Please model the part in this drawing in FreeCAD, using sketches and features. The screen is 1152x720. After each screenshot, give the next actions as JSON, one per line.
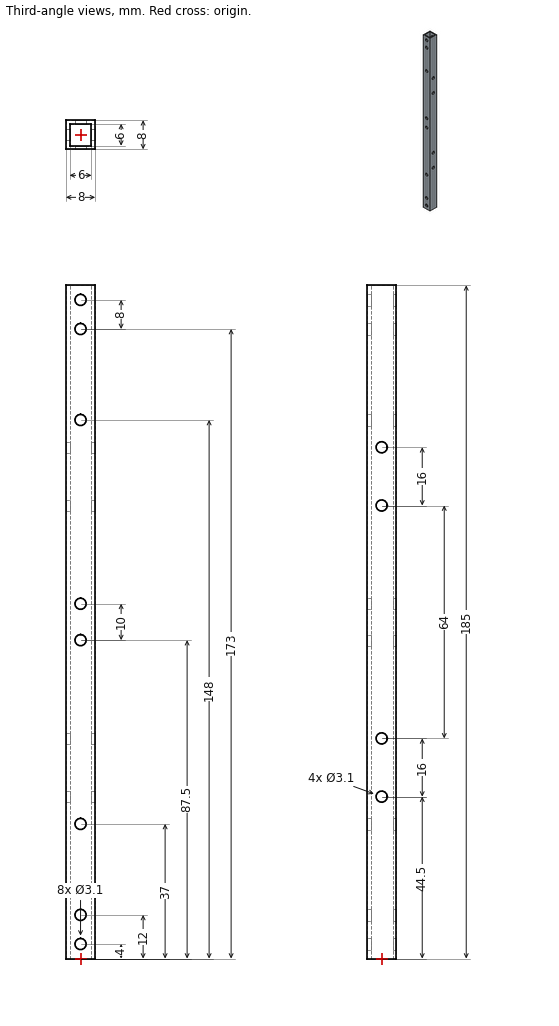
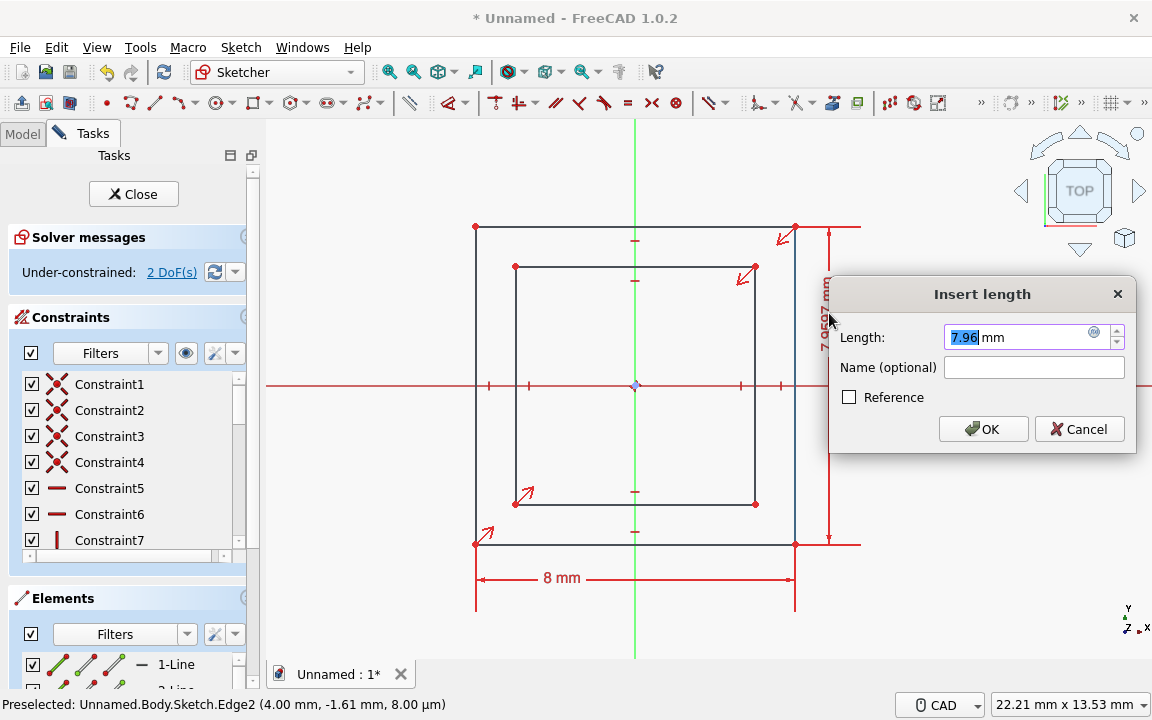
{"action": "type", "text": "8"}
{"action": "key", "text": "Return"}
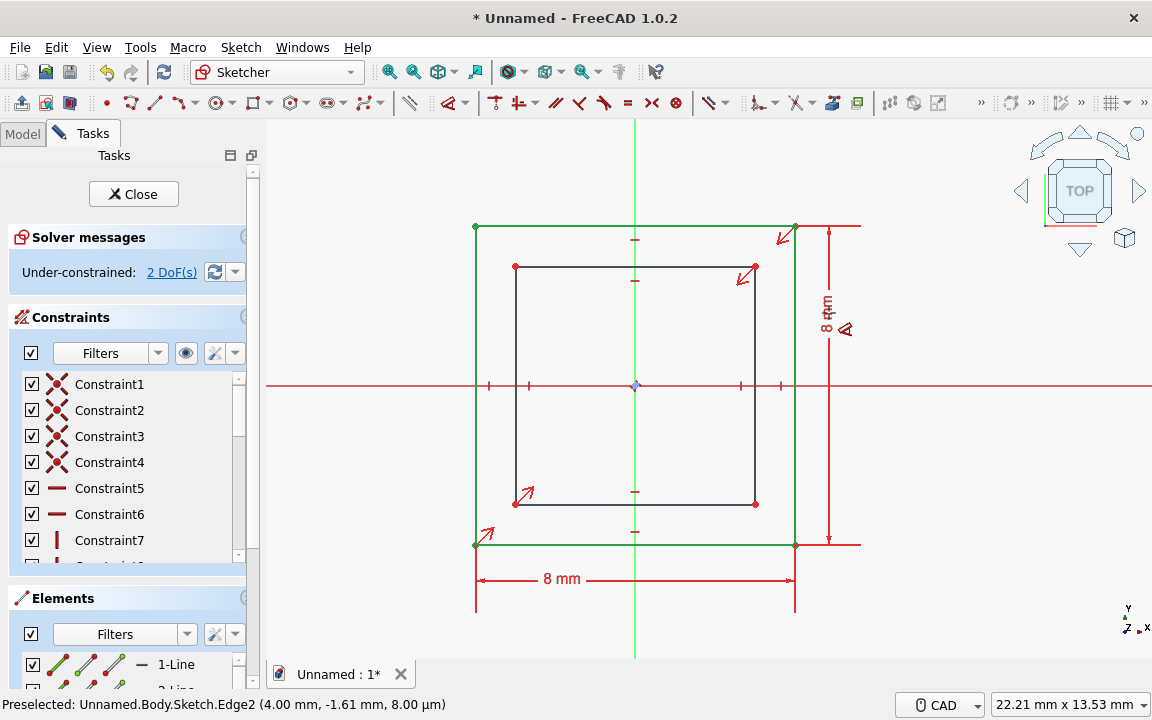
{"action": "left_click", "coordinate": [588, 505]}
{"action": "left_click", "coordinate": [580, 471]}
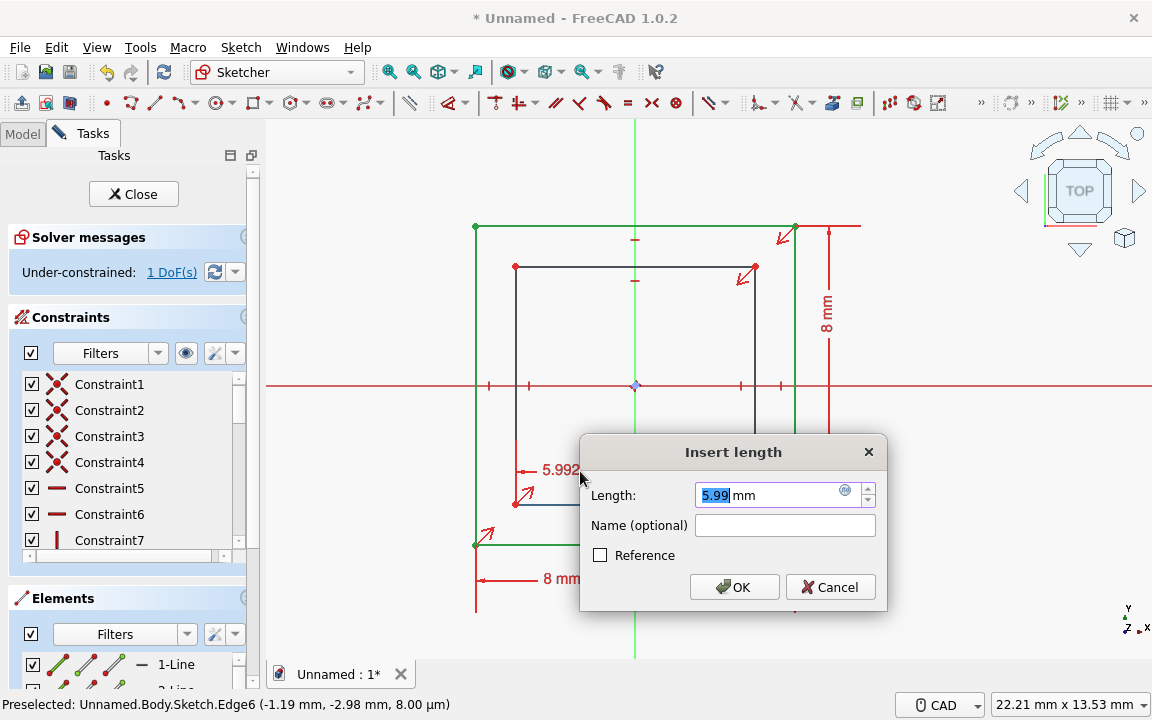
{"action": "type", "text": "6"}
{"action": "key", "text": "Return"}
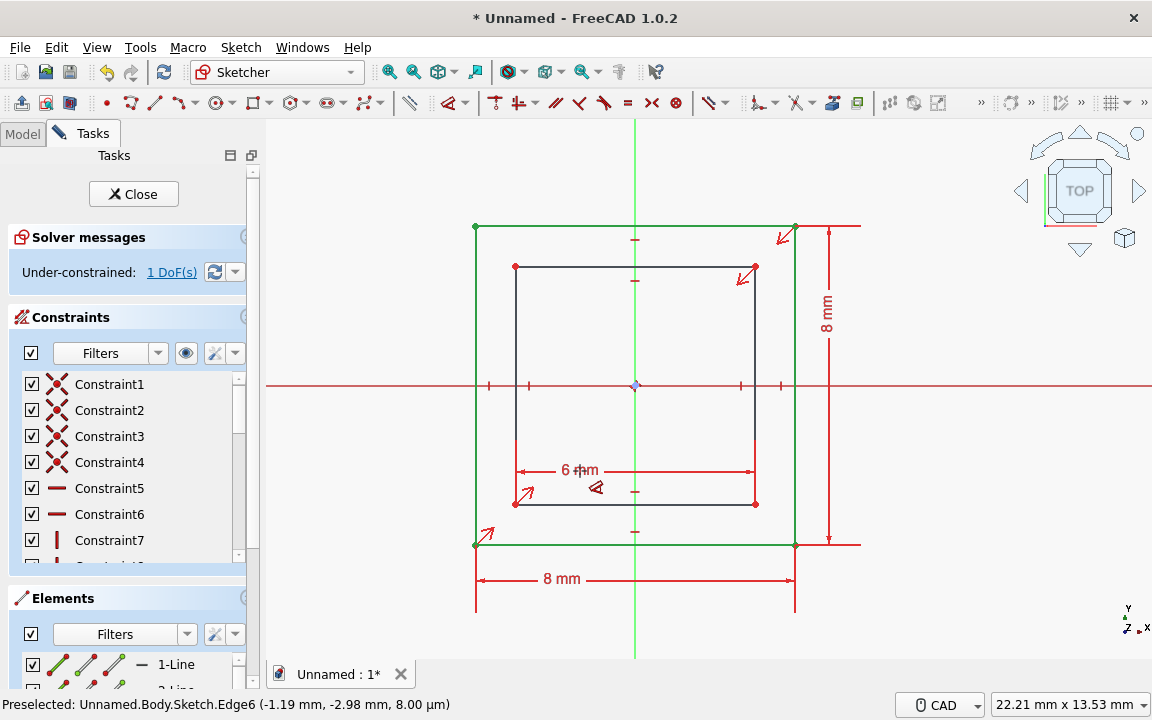
{"action": "left_click", "coordinate": [755, 433]}
{"action": "left_click", "coordinate": [721, 331]}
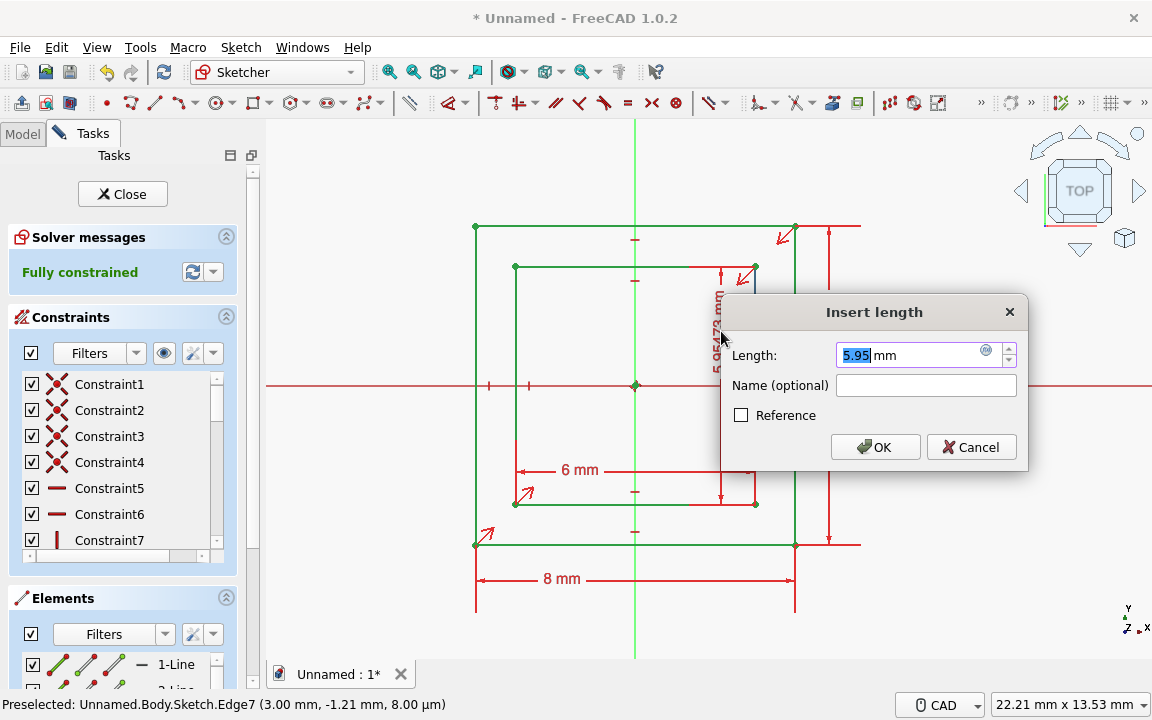
{"action": "type", "text": "6"}
{"action": "key", "text": "Return"}
{"action": "key", "text": "Escape"}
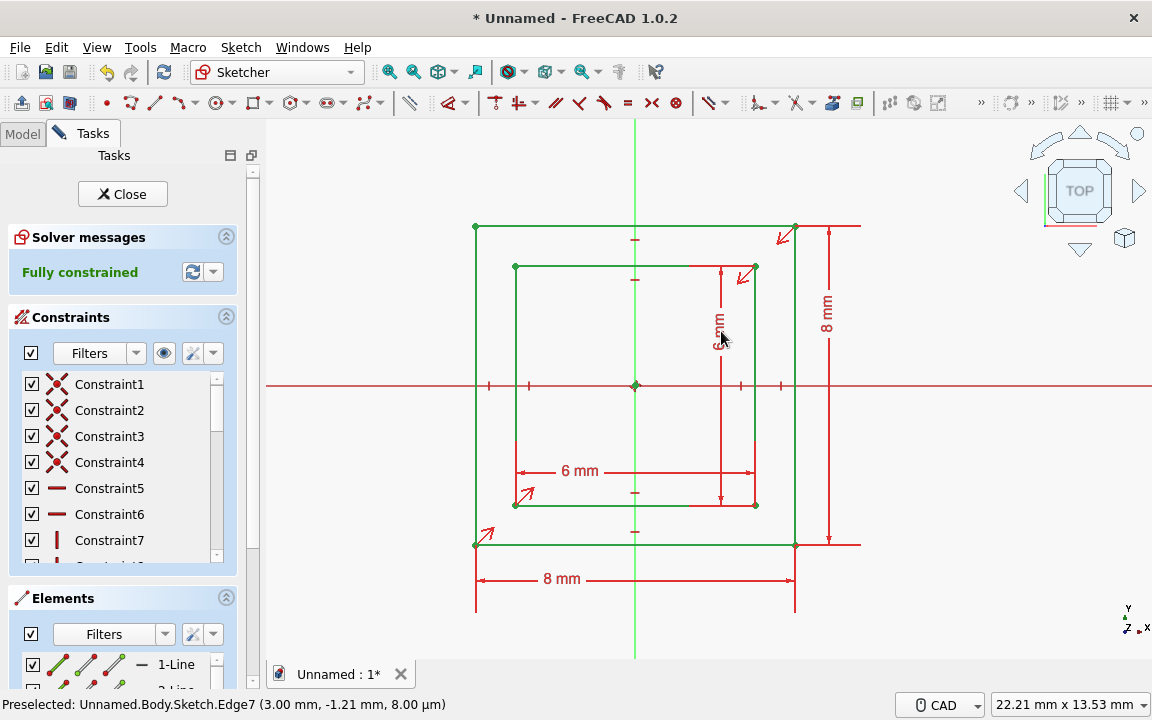
{"action": "left_click", "coordinate": [123, 194]}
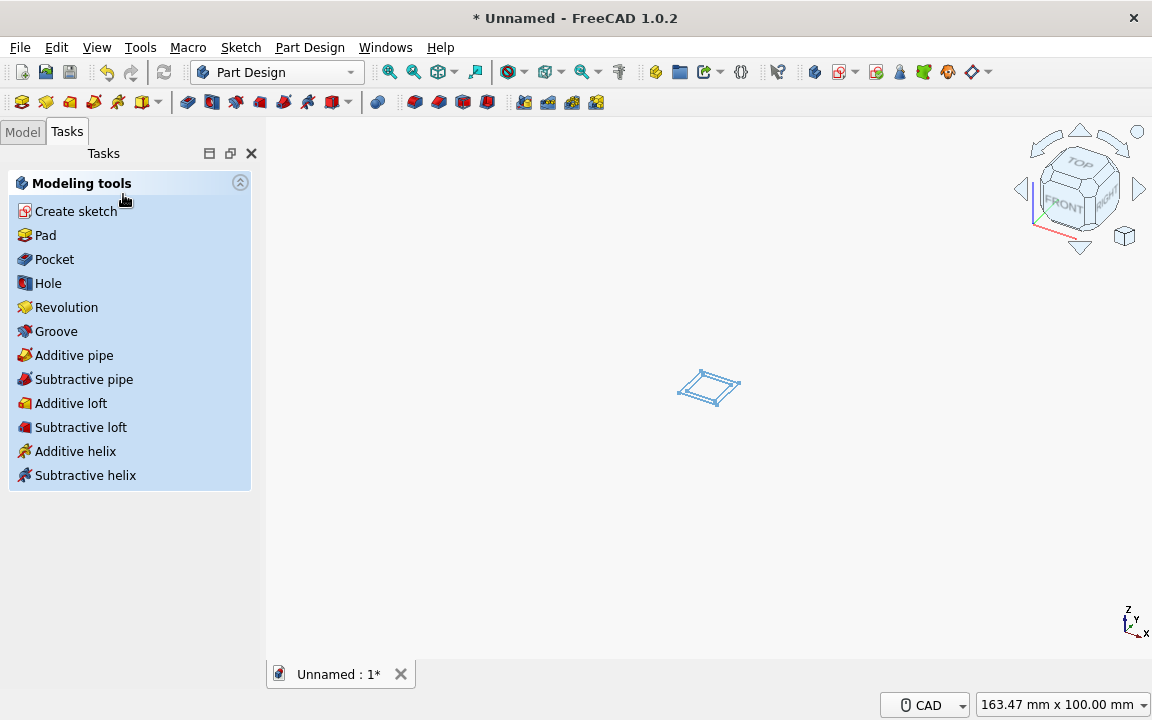
{"action": "left_click", "coordinate": [22, 102]}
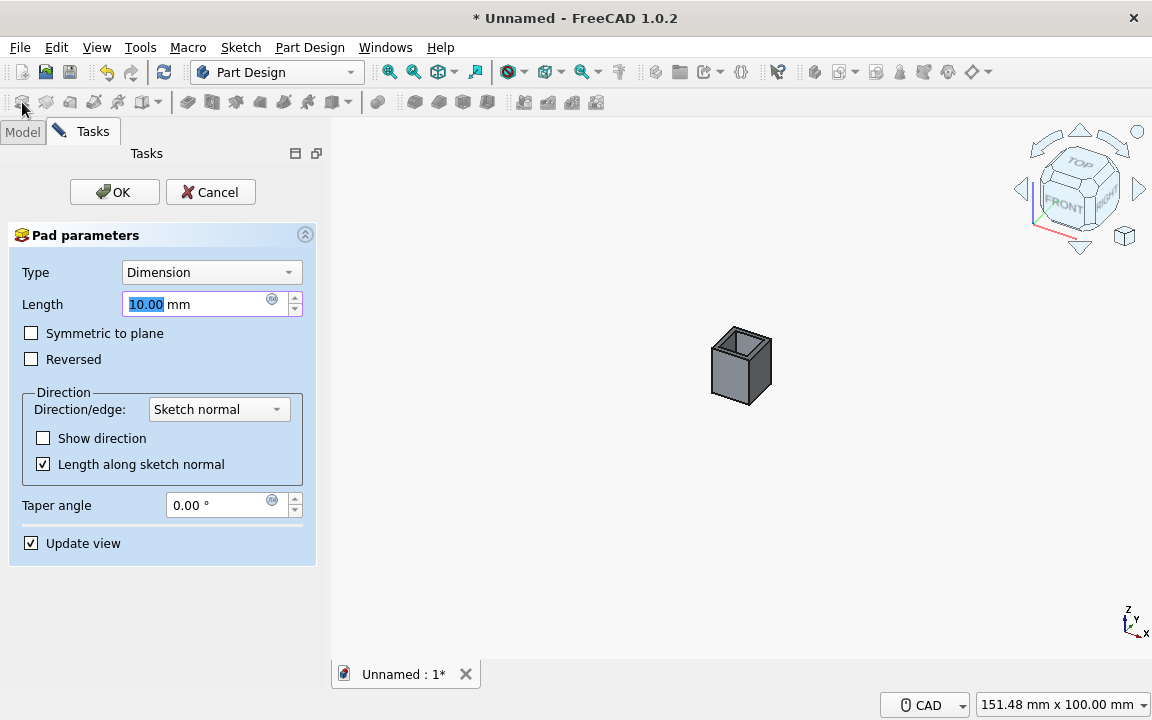
{"action": "type", "text": "185"}
{"action": "key", "text": "Tab"}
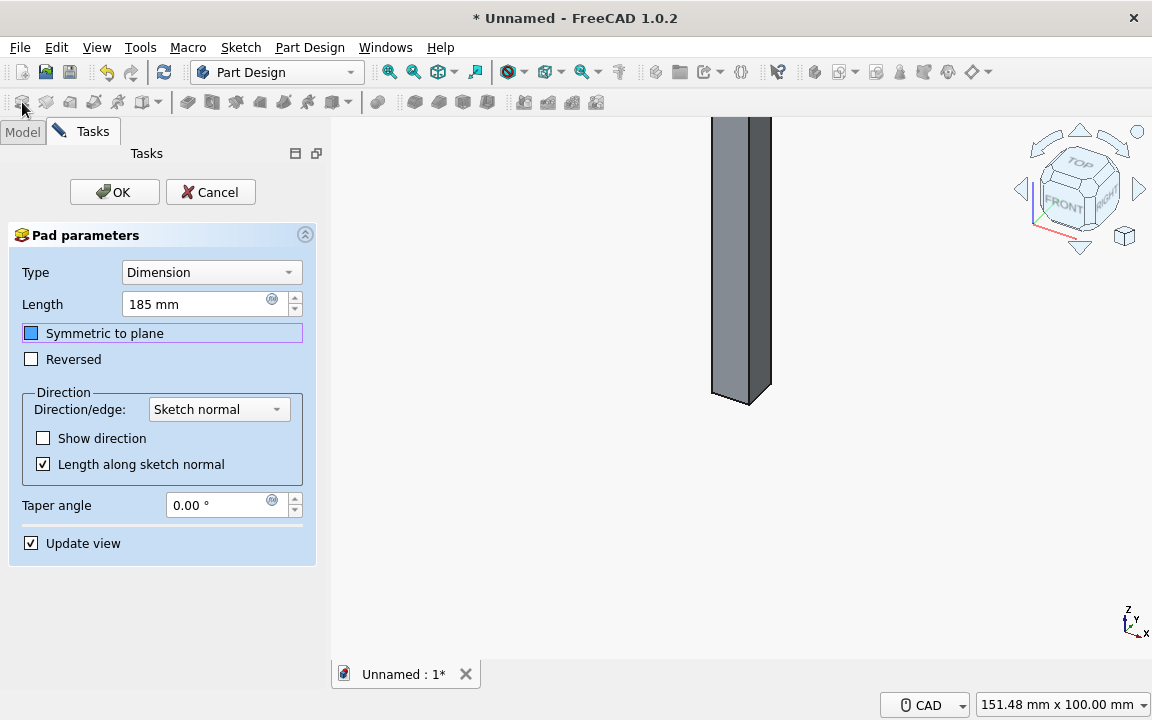
{"action": "left_click", "coordinate": [115, 192]}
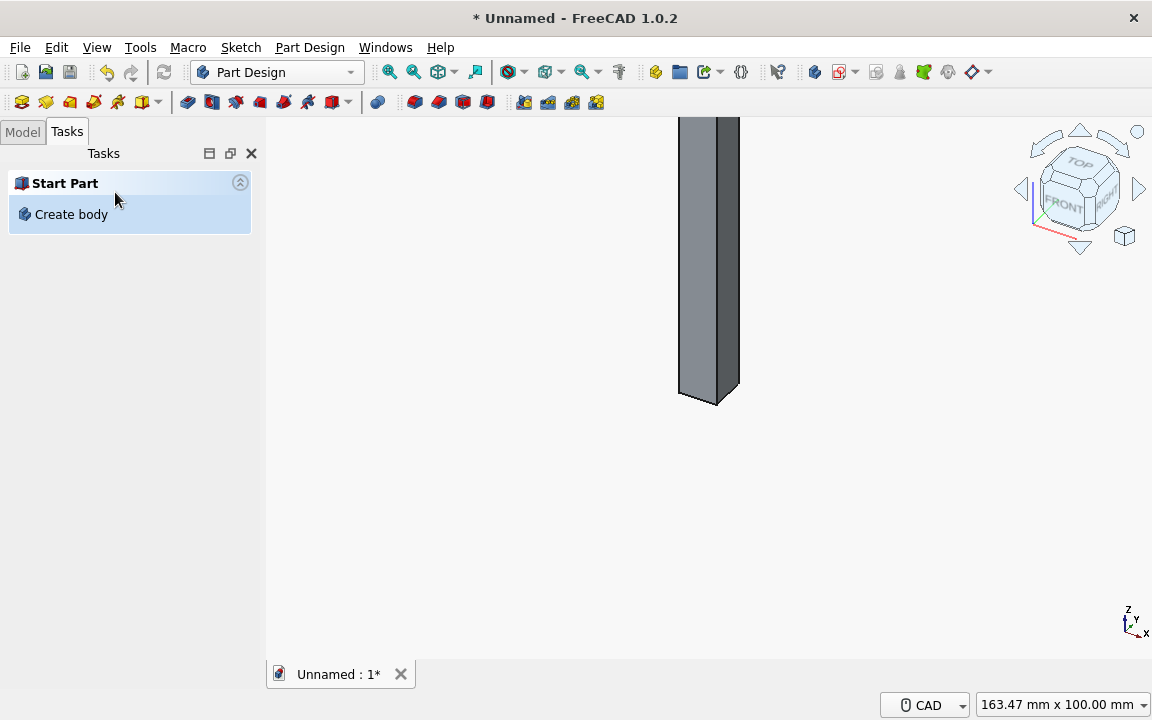
{"action": "left_click", "coordinate": [390, 72]}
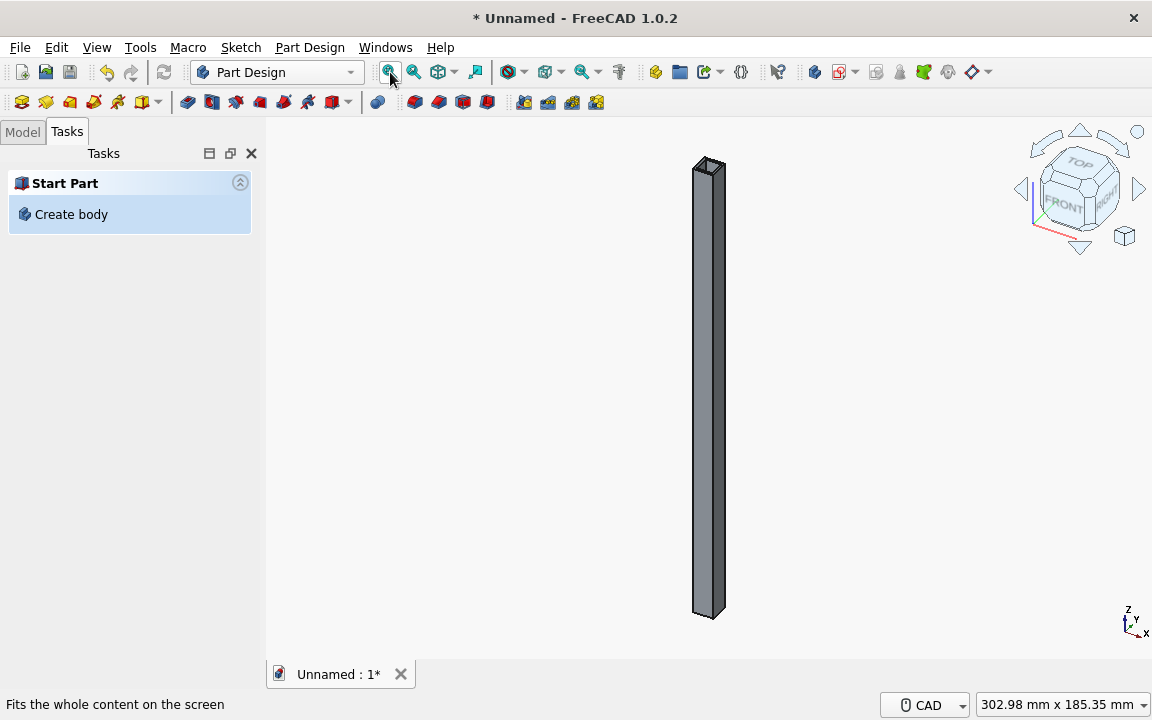
{"action": "key", "text": "0"}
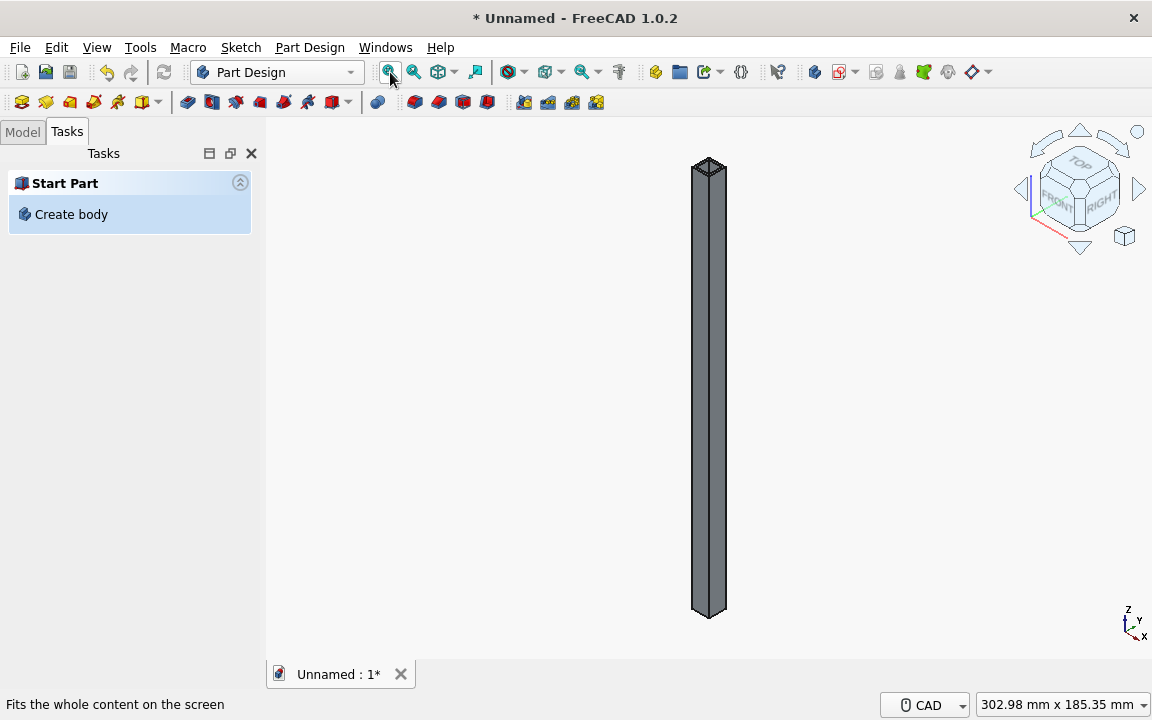
{"action": "left_click", "coordinate": [717, 202]}